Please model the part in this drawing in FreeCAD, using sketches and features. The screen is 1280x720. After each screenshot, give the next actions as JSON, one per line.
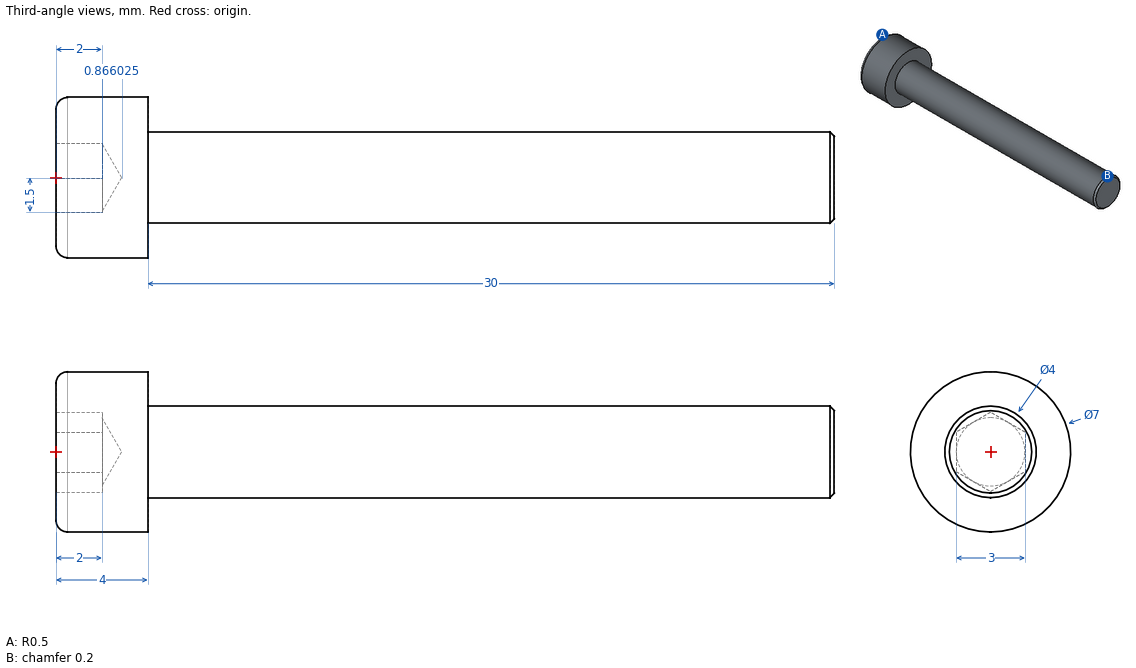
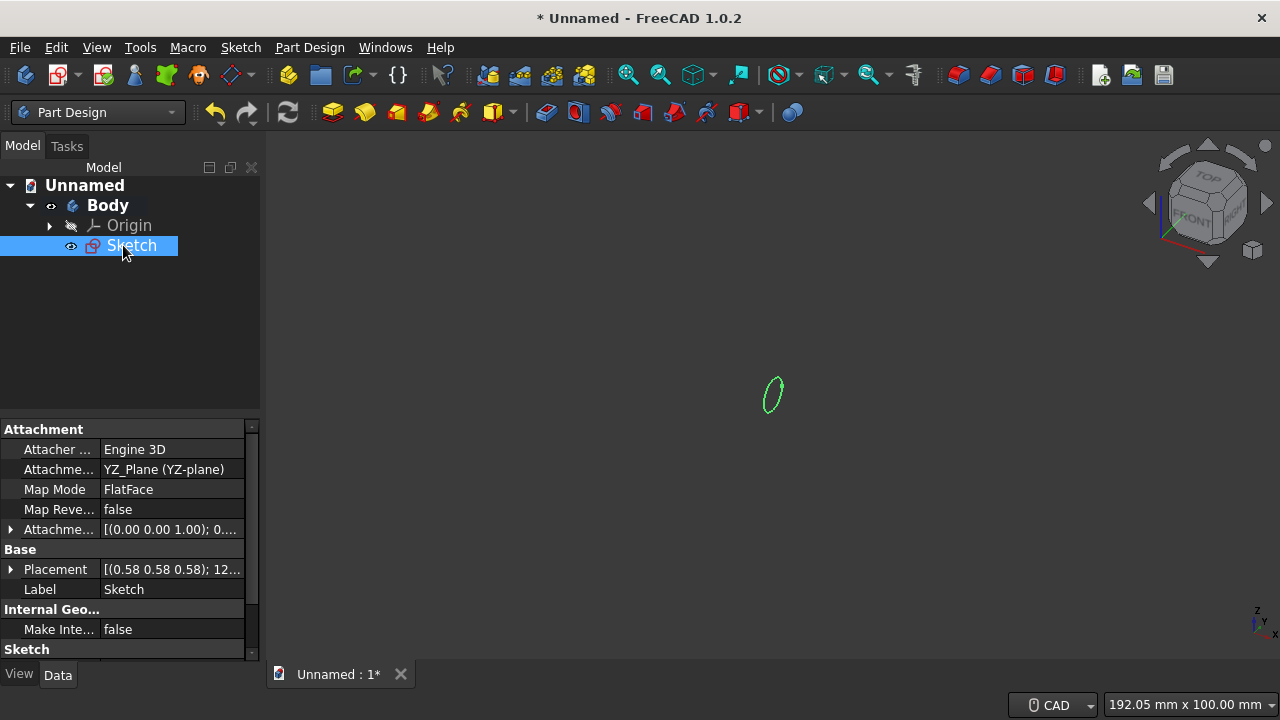
{"action": "left_click", "coordinate": [334, 112]}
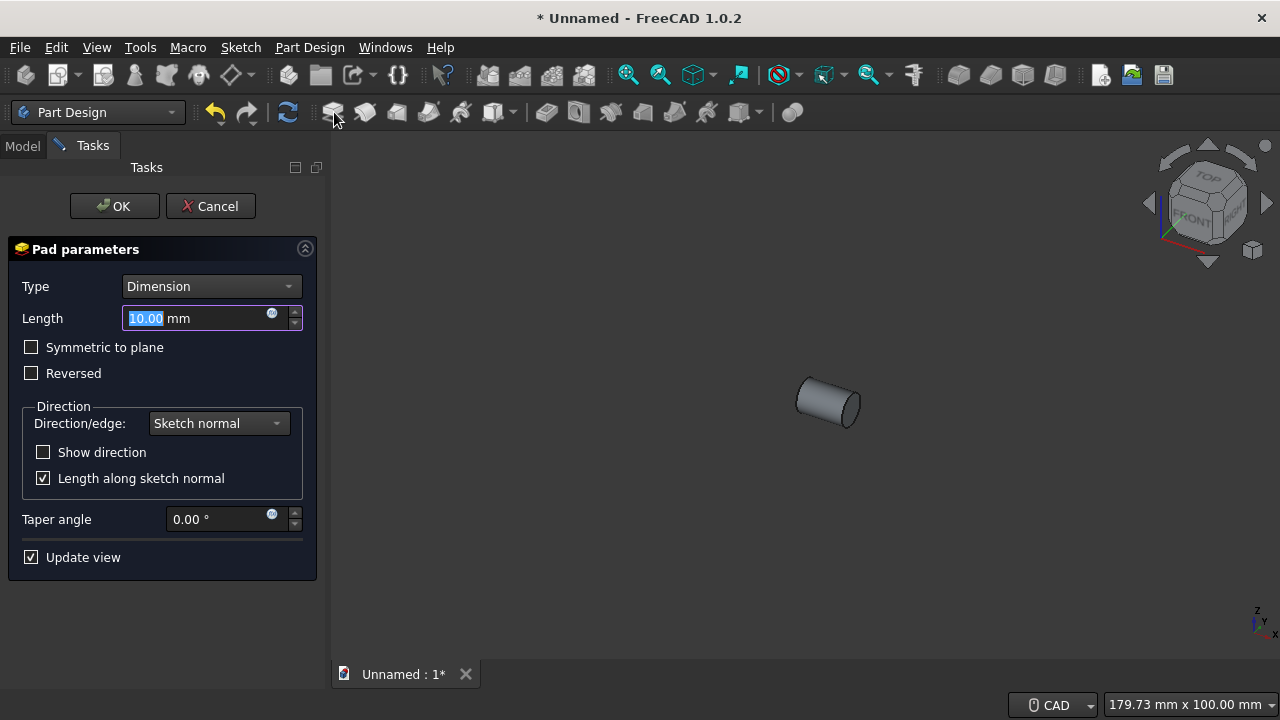
{"action": "type", "text": "4"}
{"action": "key", "text": "Tab"}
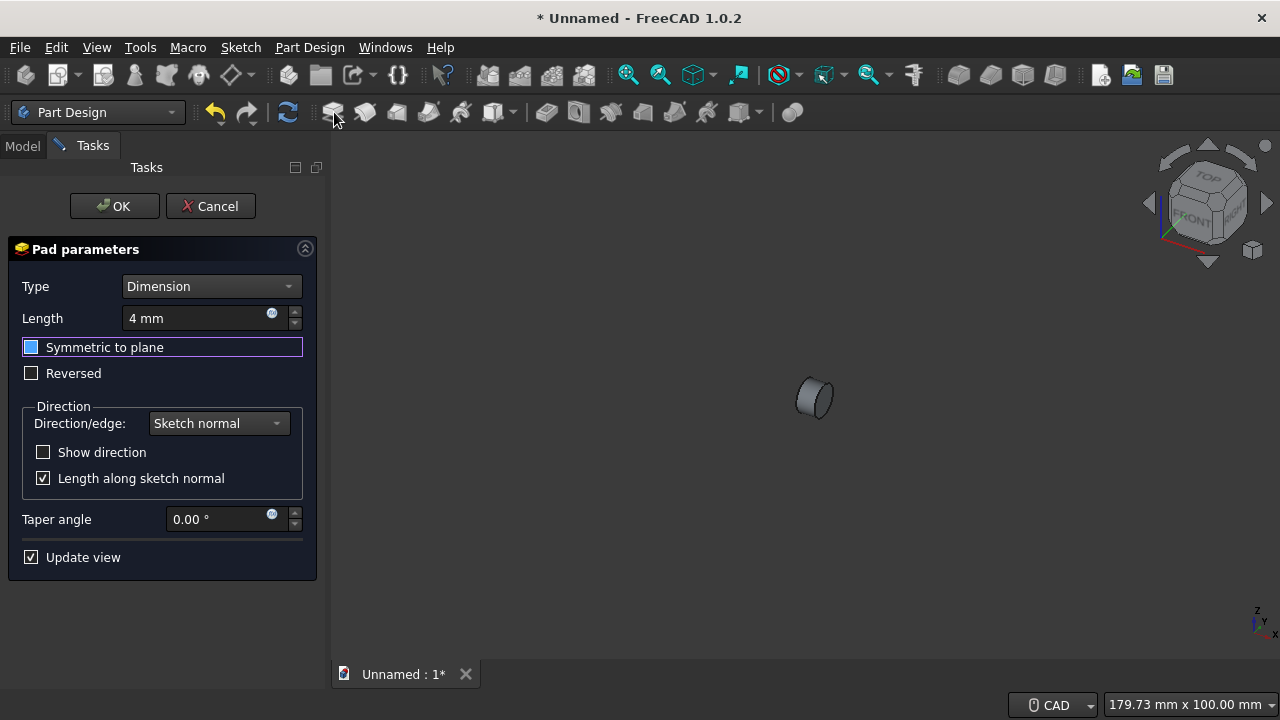
{"action": "left_click", "coordinate": [115, 206]}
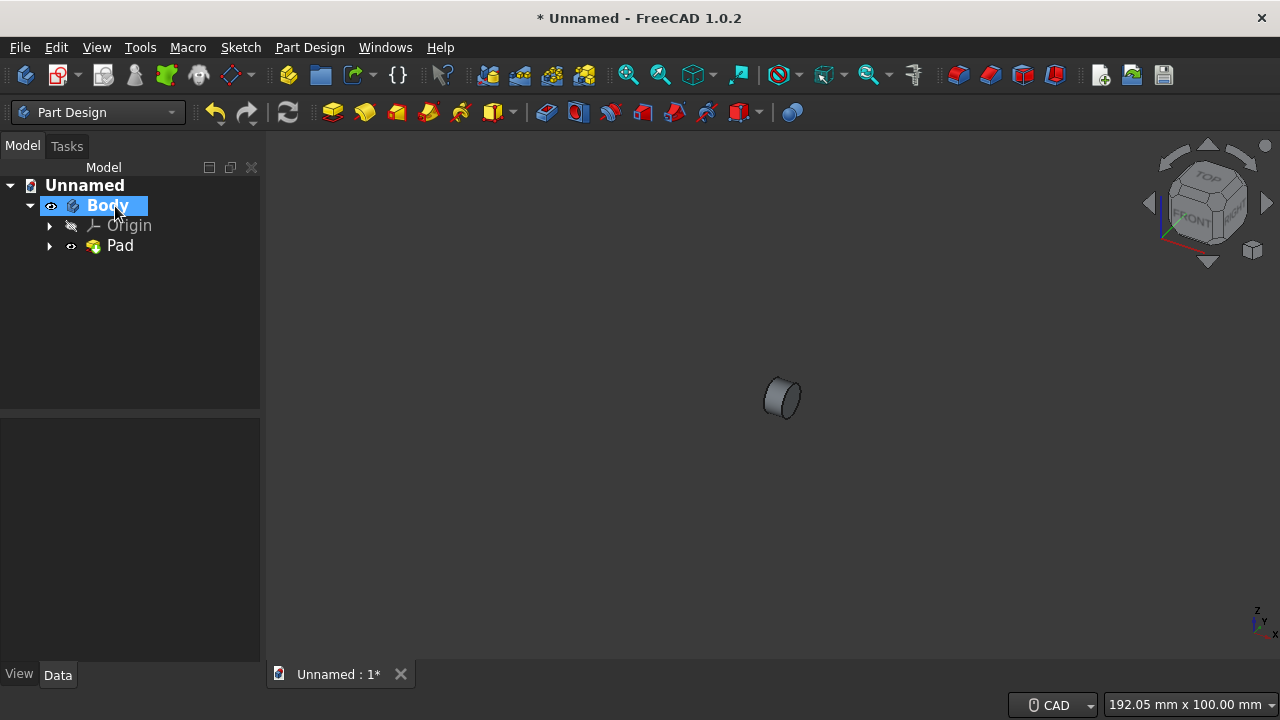
{"action": "left_click", "coordinate": [630, 76]}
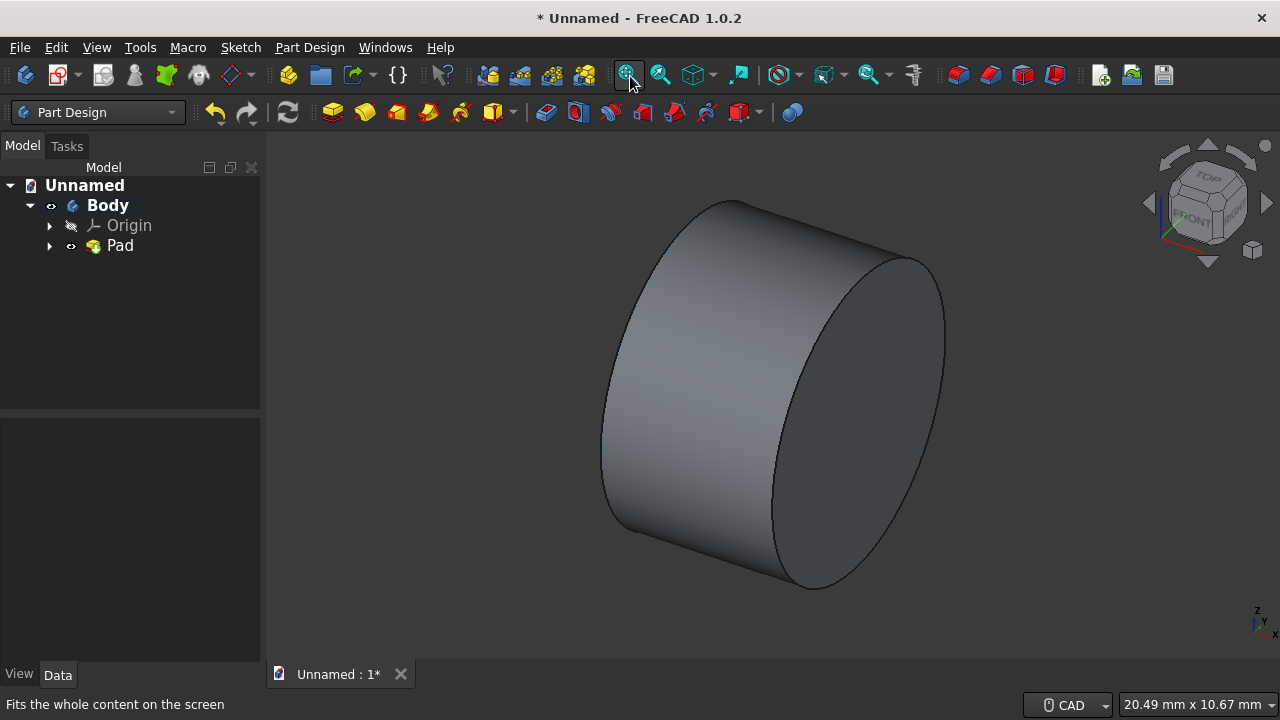
{"action": "left_click", "coordinate": [859, 422]}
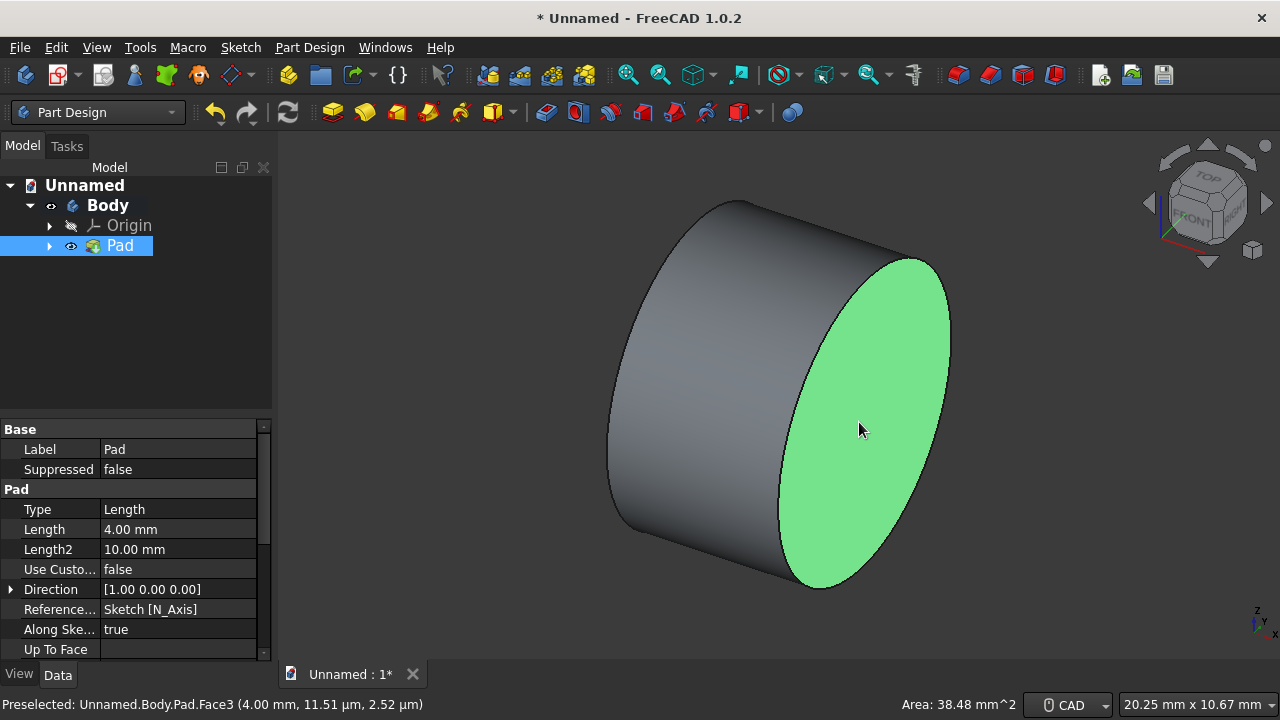
{"action": "left_click", "coordinate": [58, 76]}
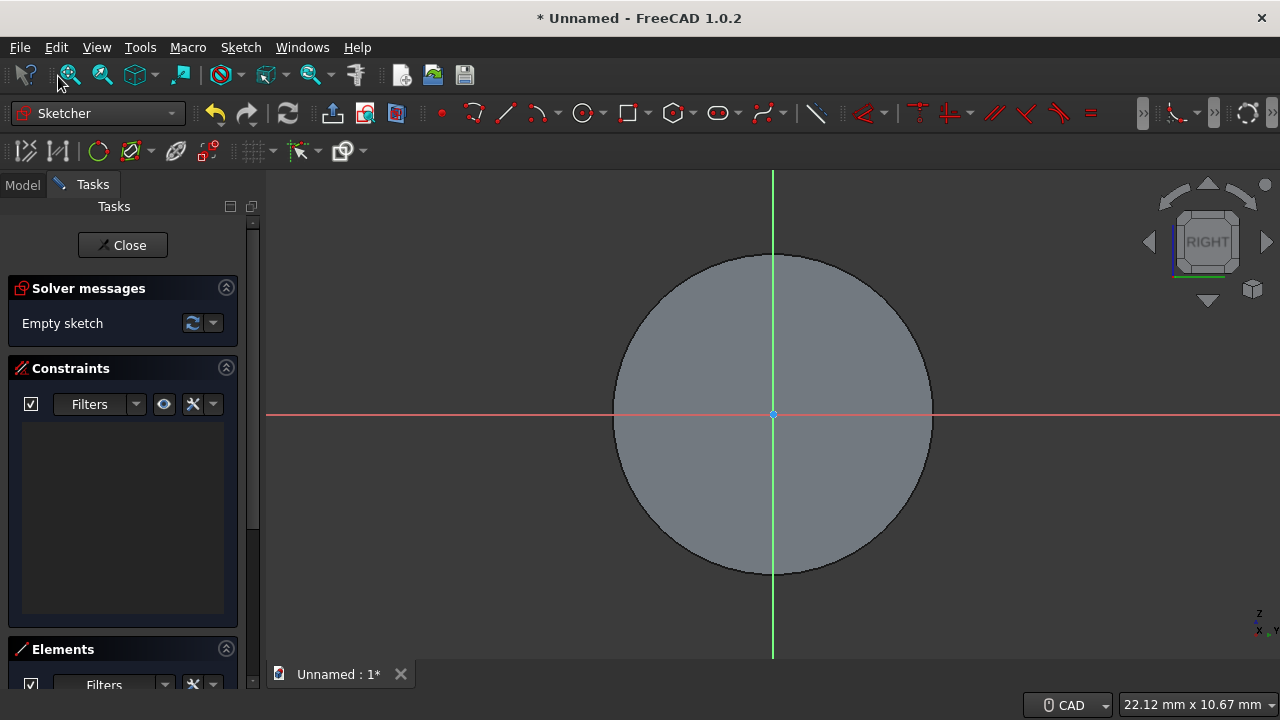
{"action": "scroll", "coordinate": [856, 415], "scroll_direction": "up", "scroll_amount": 3}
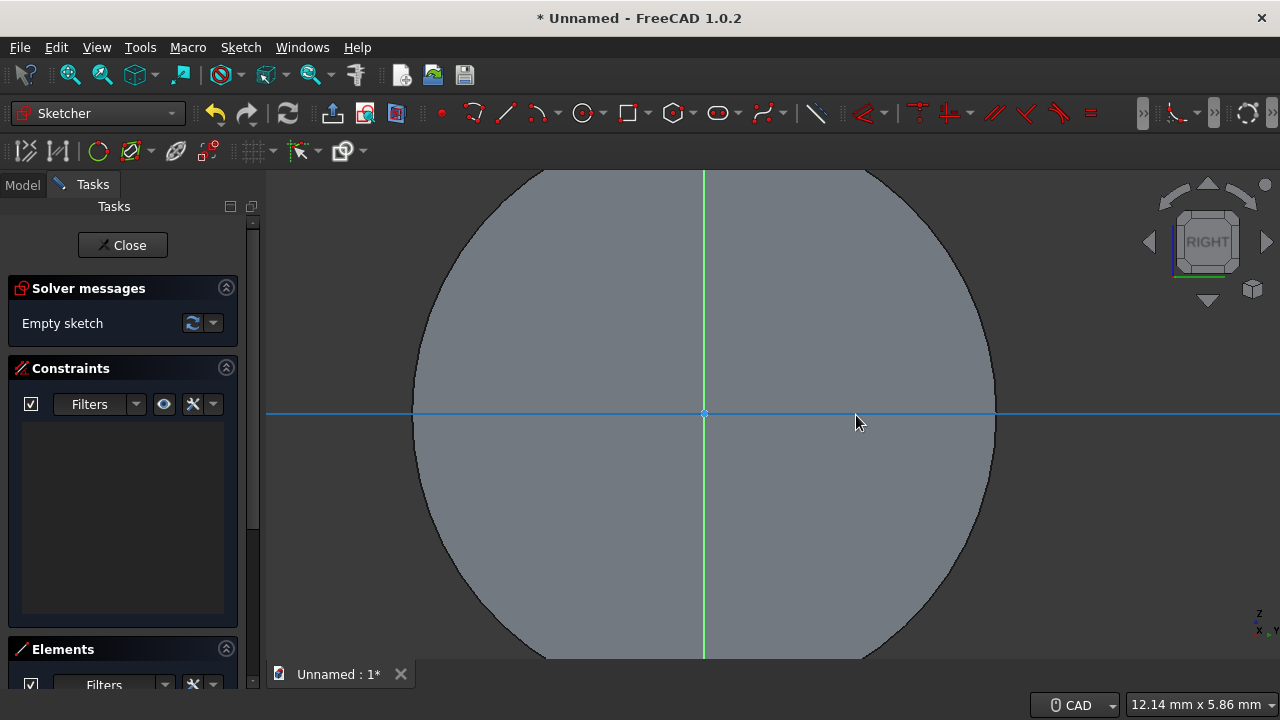
{"action": "left_click", "coordinate": [584, 114]}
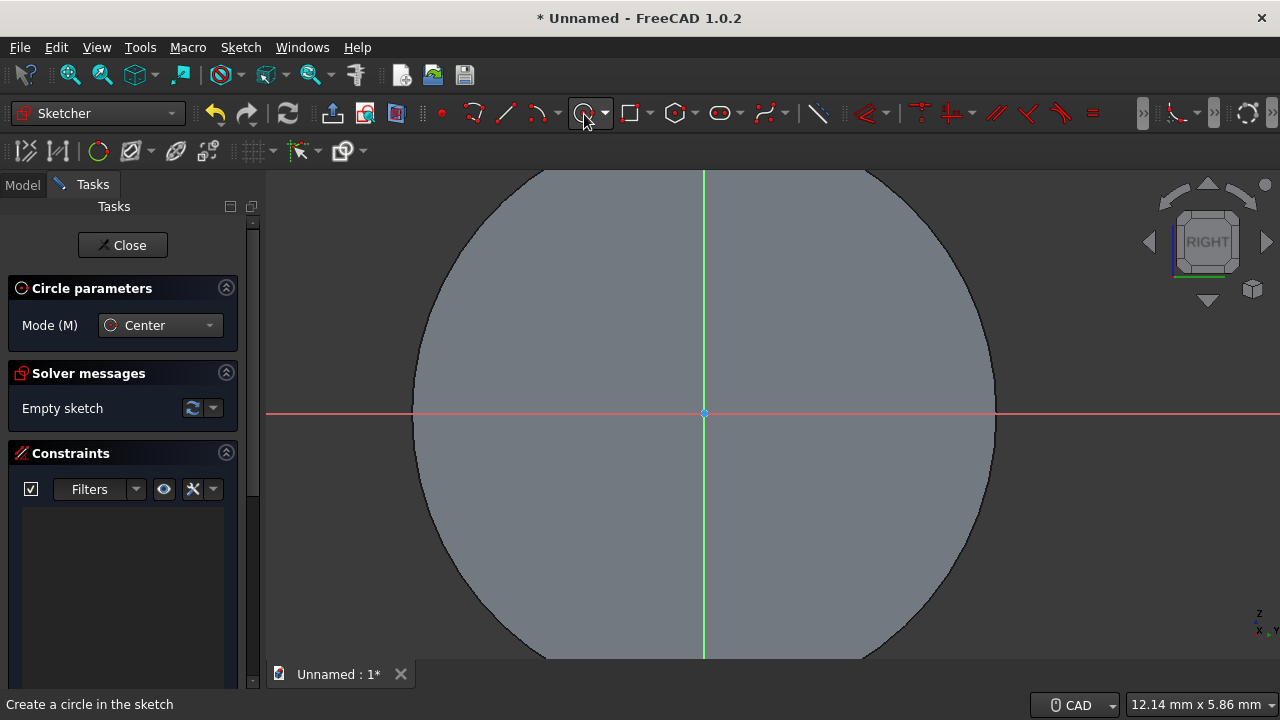
{"action": "left_click", "coordinate": [704, 414]}
{"action": "left_click", "coordinate": [822, 296]}
{"action": "key", "text": "Escape"}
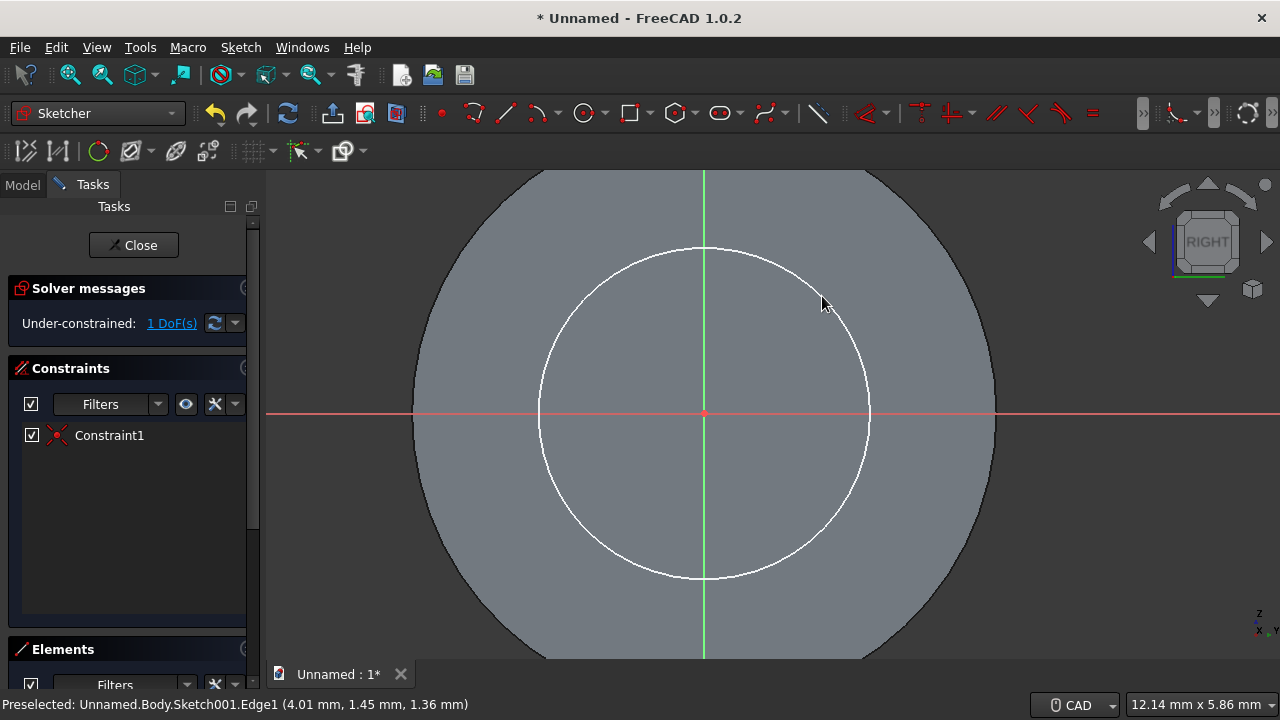
{"action": "left_click", "coordinate": [866, 114]}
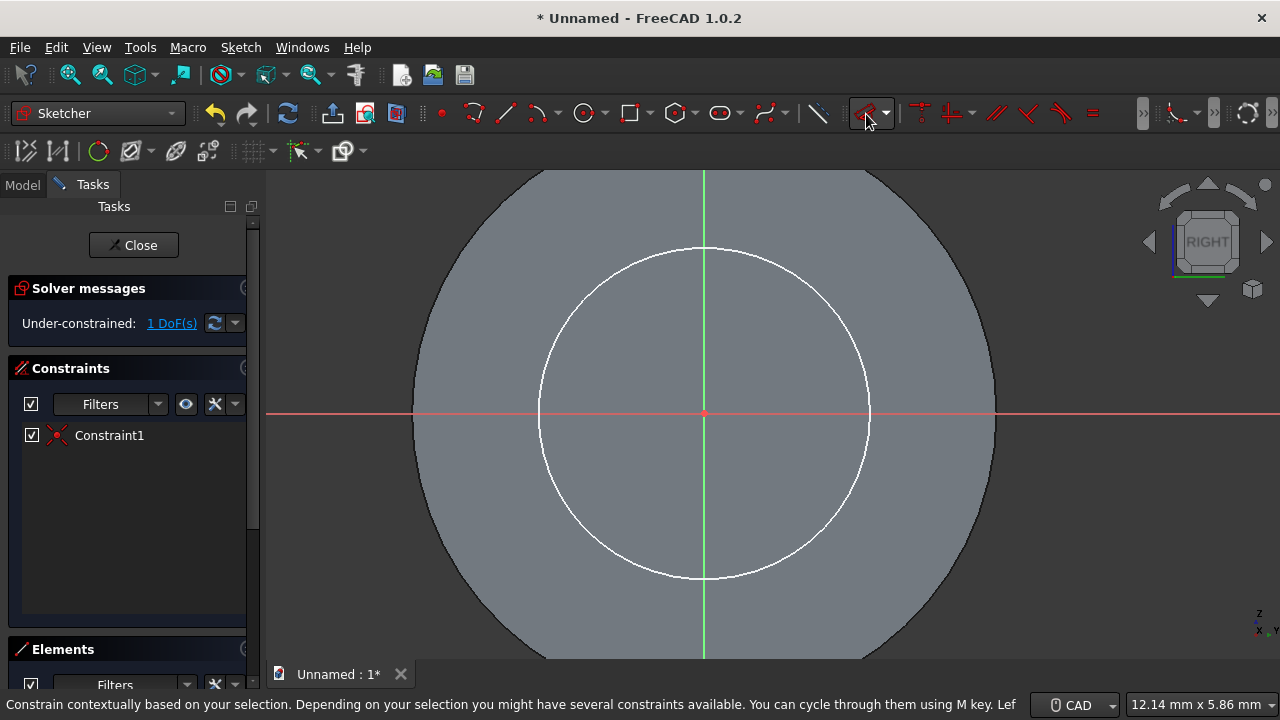
{"action": "left_click", "coordinate": [821, 296]}
{"action": "left_click", "coordinate": [844, 273]}